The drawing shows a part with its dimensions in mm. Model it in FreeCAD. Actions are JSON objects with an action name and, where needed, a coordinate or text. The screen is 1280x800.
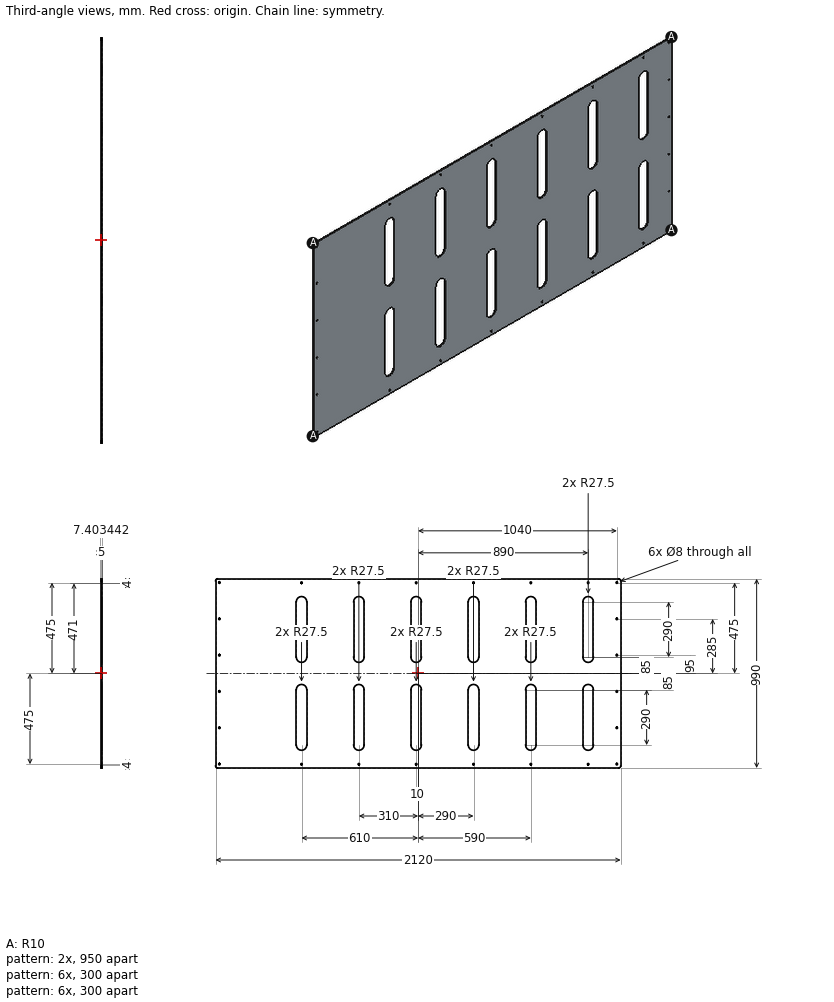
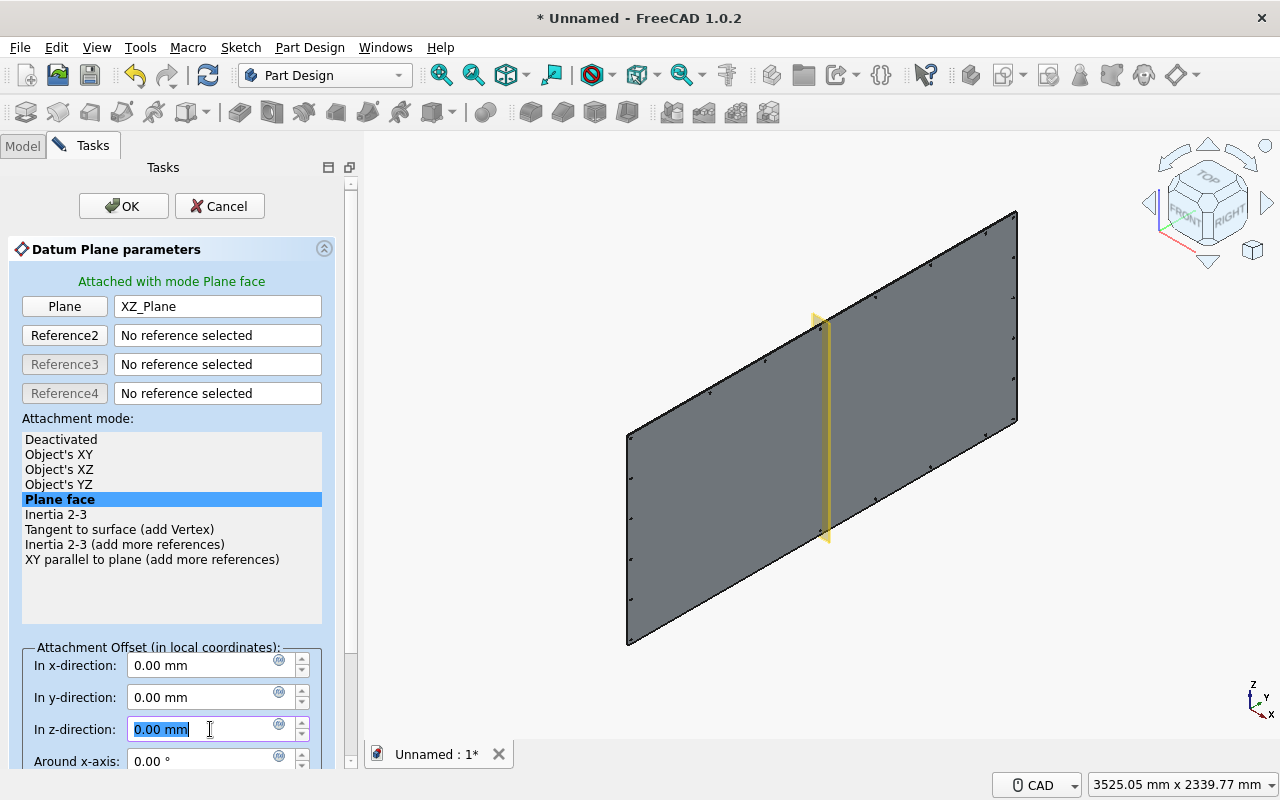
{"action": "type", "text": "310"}
{"action": "key", "text": "Tab"}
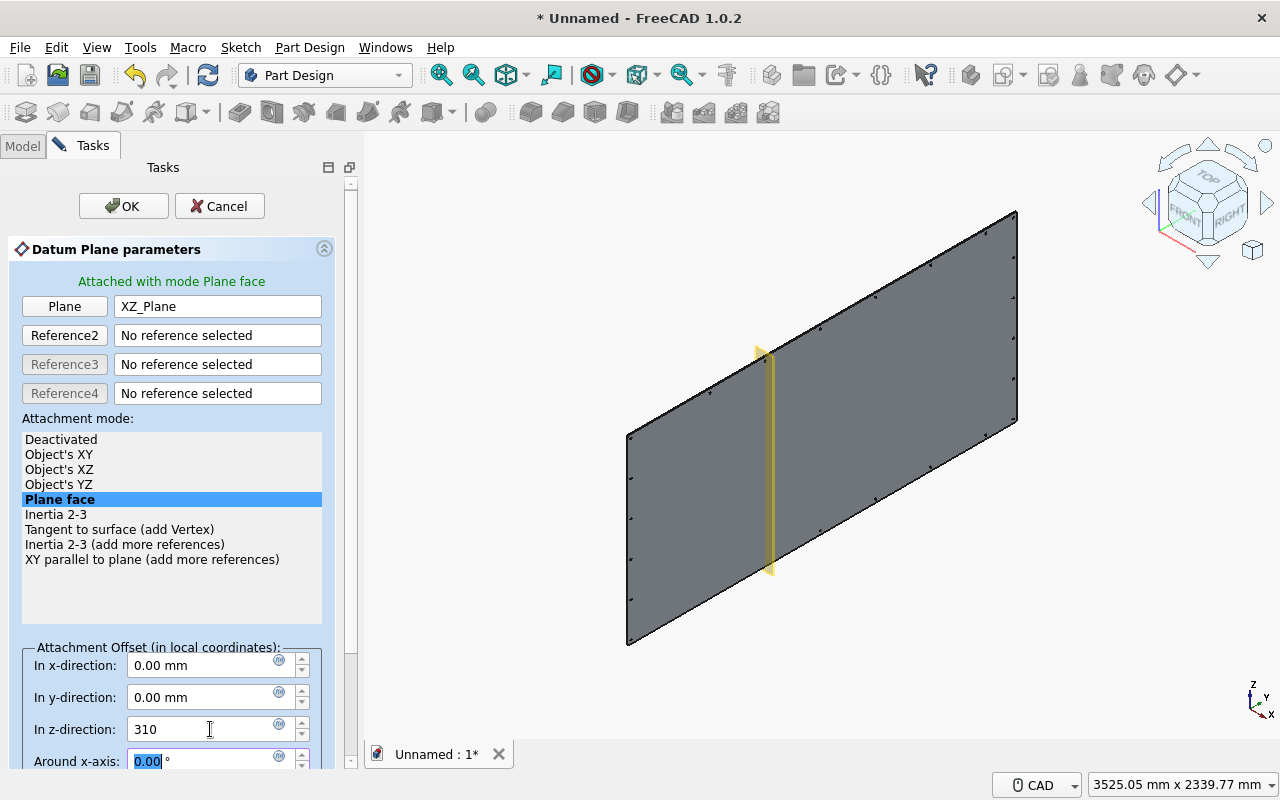
{"action": "left_click", "coordinate": [124, 206]}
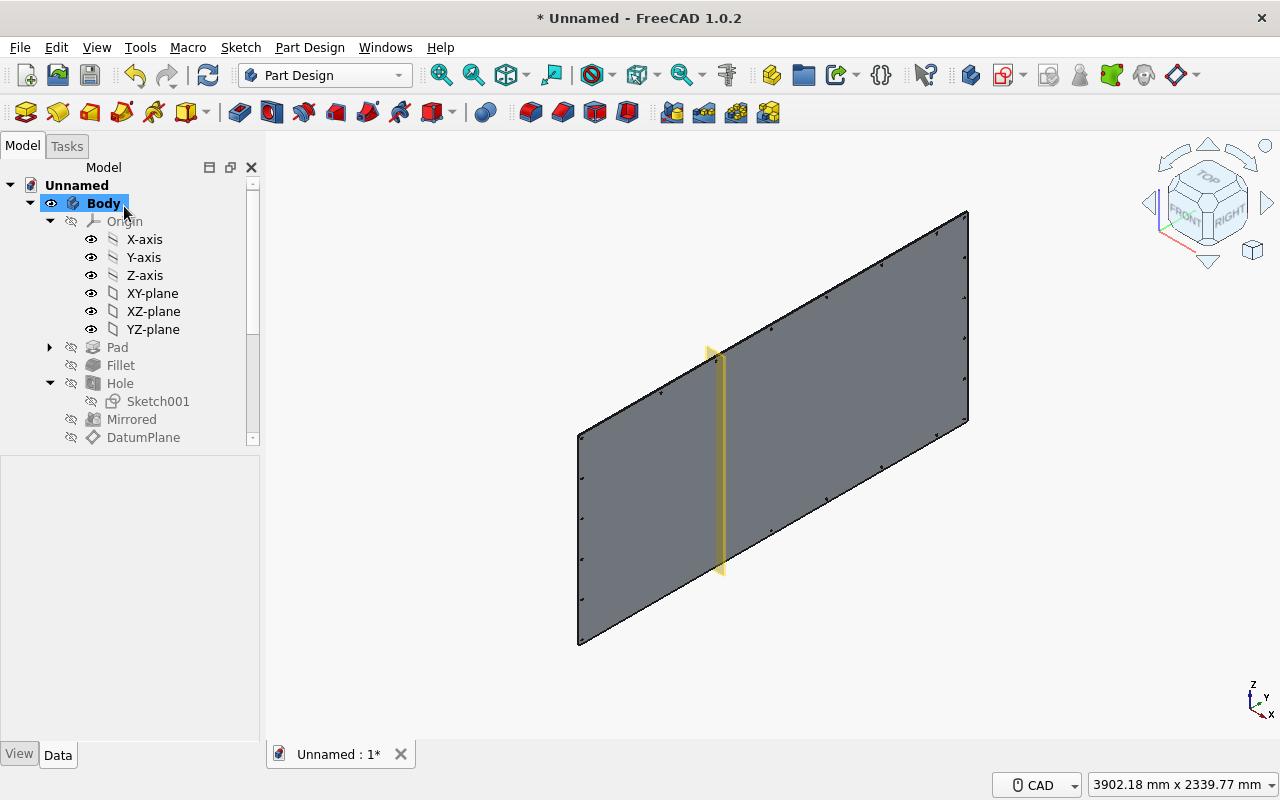
{"action": "scroll", "coordinate": [100, 307], "scroll_direction": "down", "scroll_amount": 3}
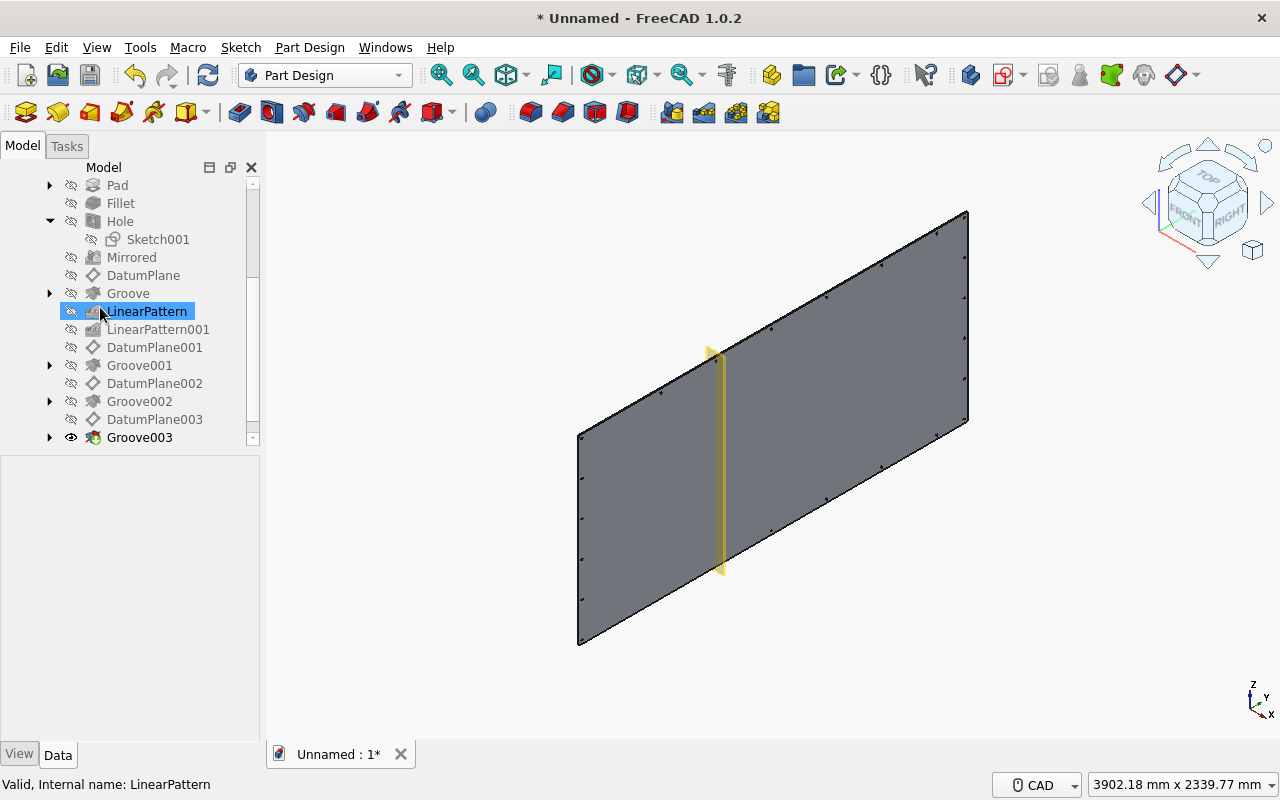
{"action": "scroll", "coordinate": [140, 307], "scroll_direction": "up", "scroll_amount": 15}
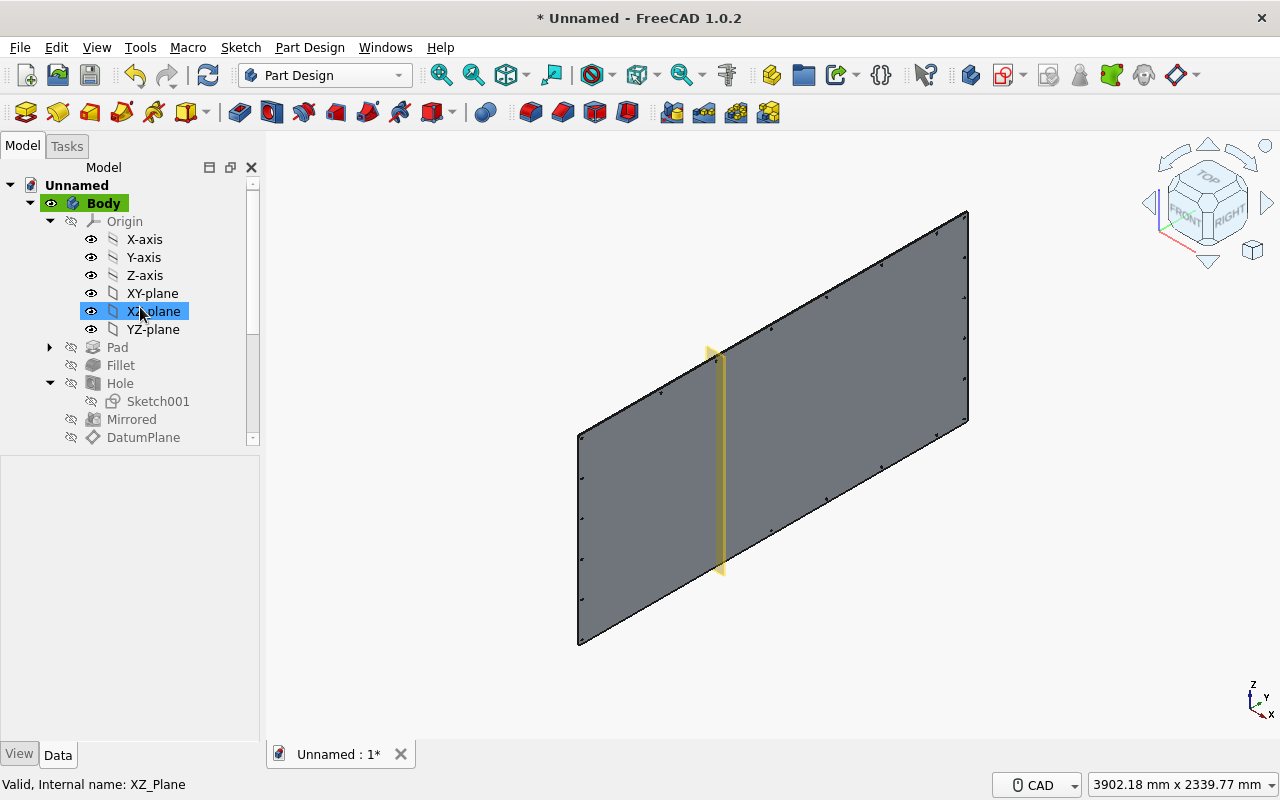
{"action": "scroll", "coordinate": [100, 307], "scroll_direction": "down", "scroll_amount": 6}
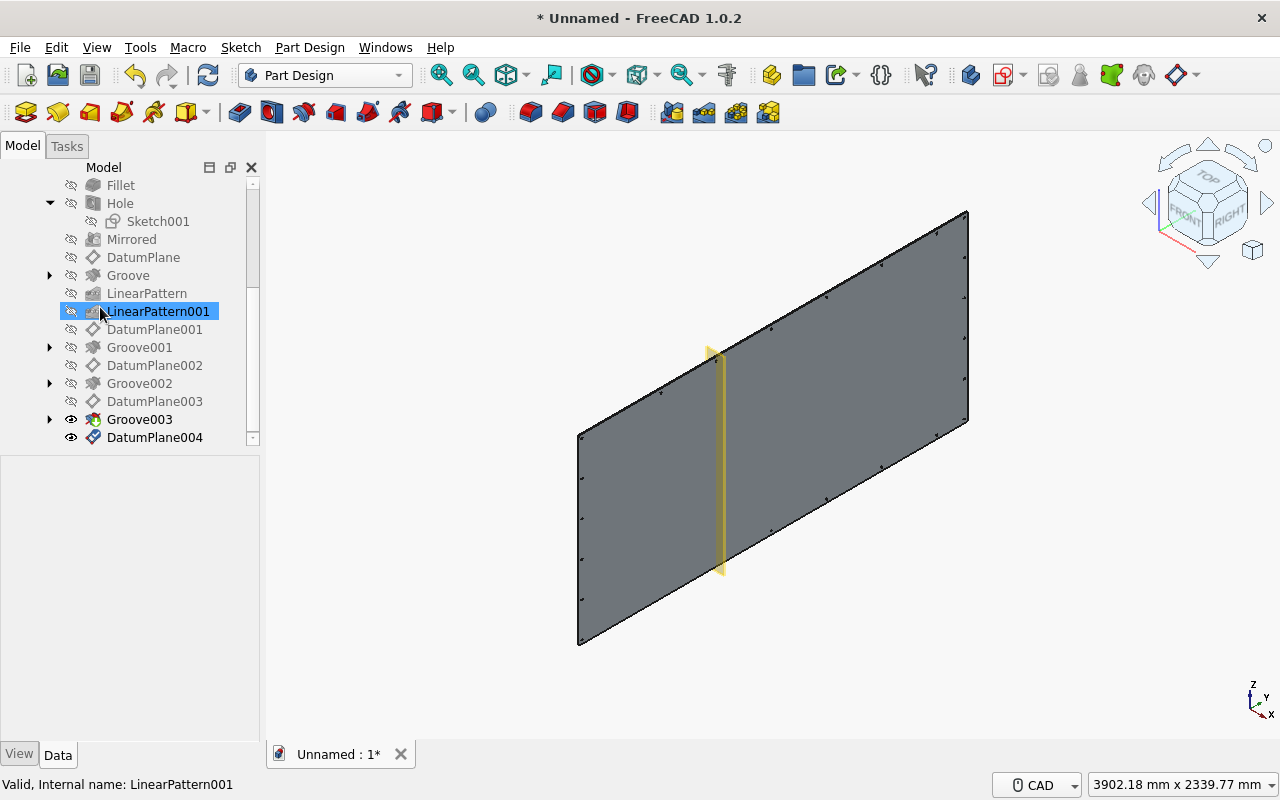
{"action": "left_click", "coordinate": [116, 437]}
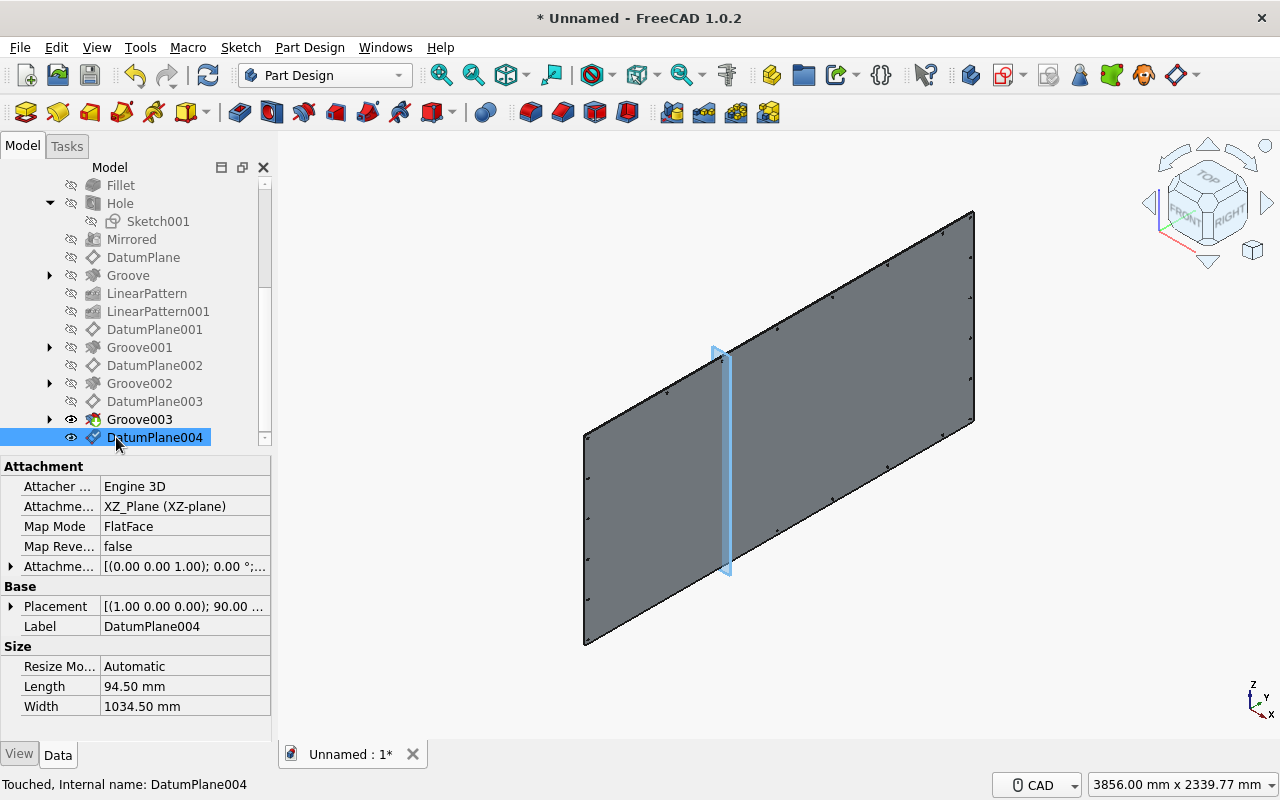
{"action": "left_click", "coordinate": [1004, 76]}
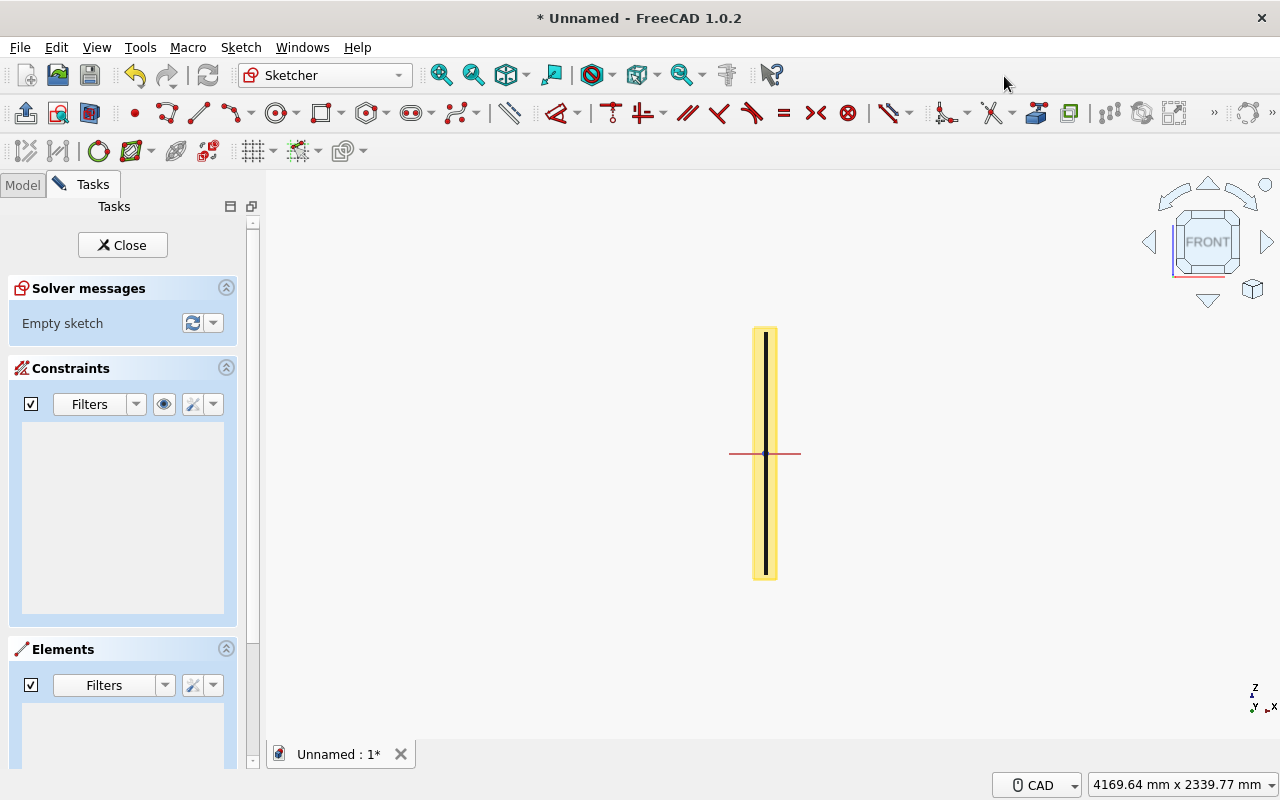
{"action": "left_click", "coordinate": [90, 114]}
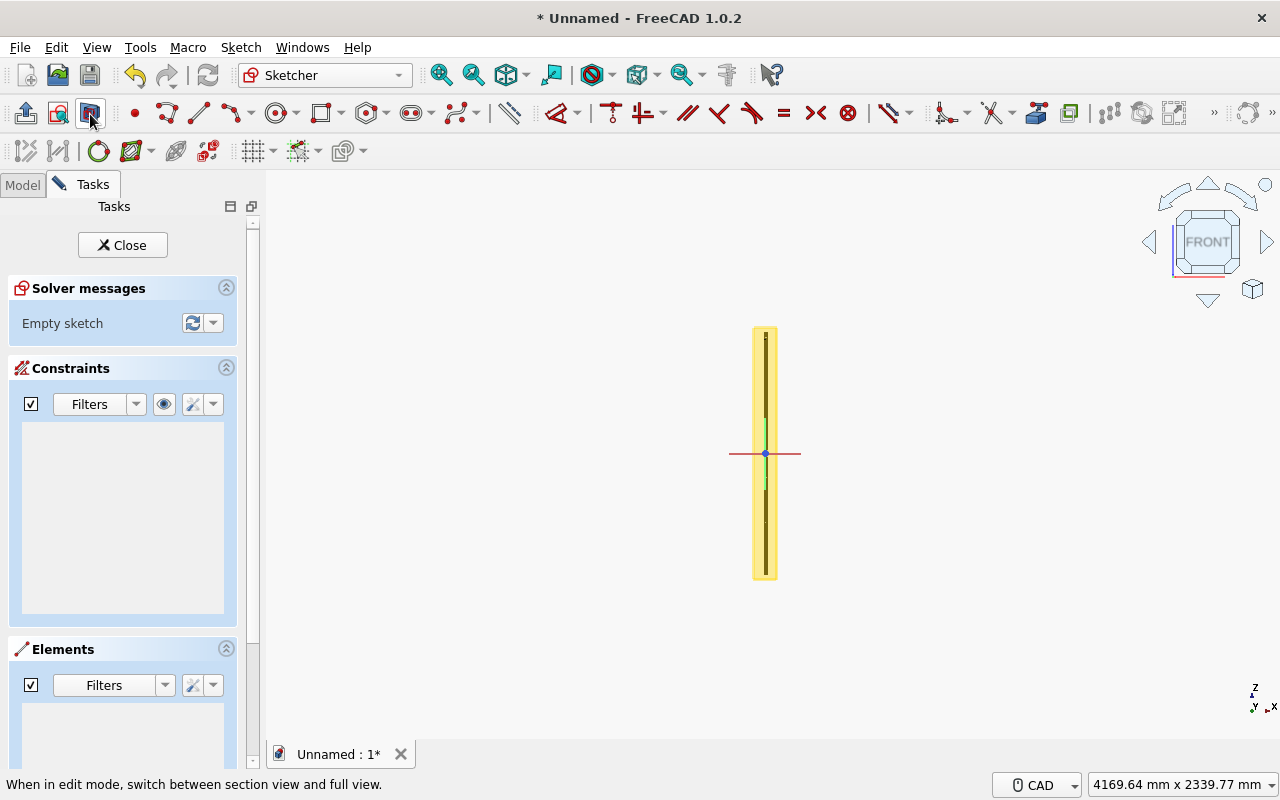
{"action": "scroll", "coordinate": [769, 576], "scroll_direction": "up", "scroll_amount": 15}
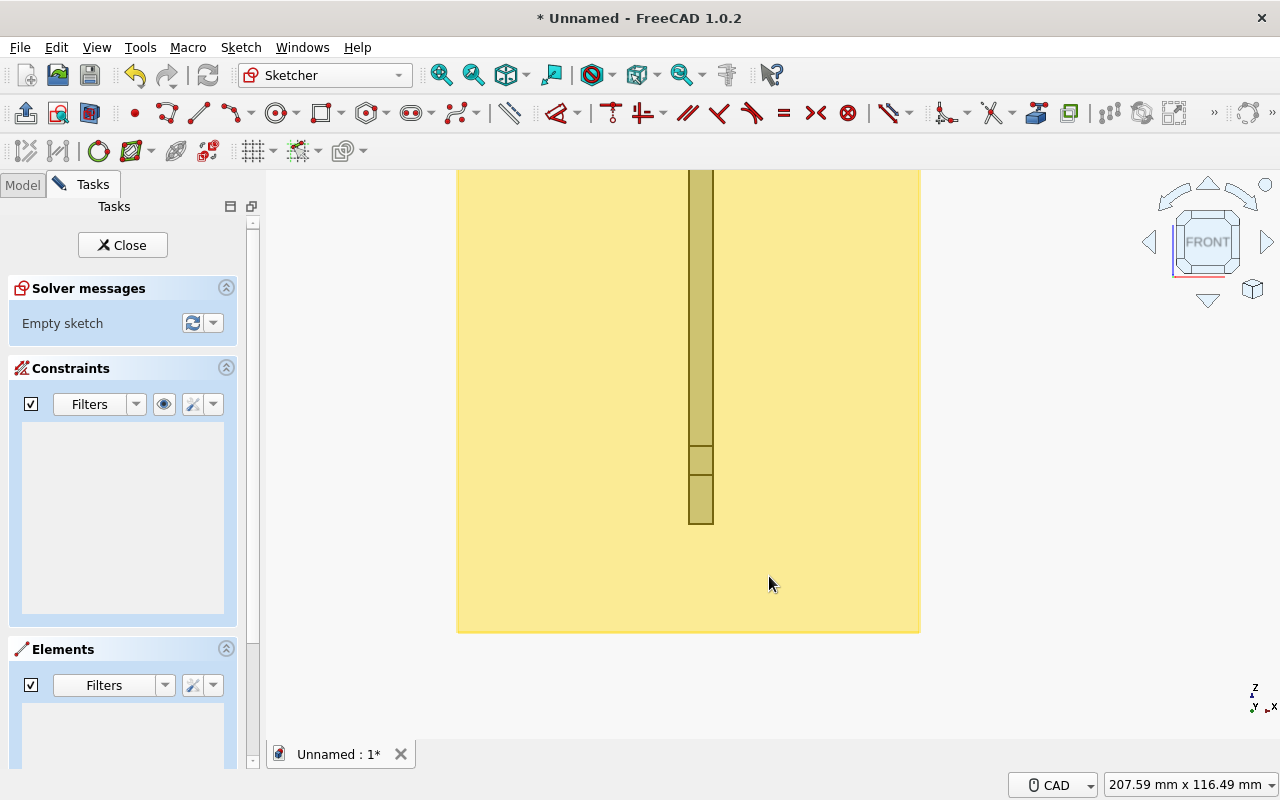
{"action": "scroll", "coordinate": [686, 434], "scroll_direction": "up", "scroll_amount": 12}